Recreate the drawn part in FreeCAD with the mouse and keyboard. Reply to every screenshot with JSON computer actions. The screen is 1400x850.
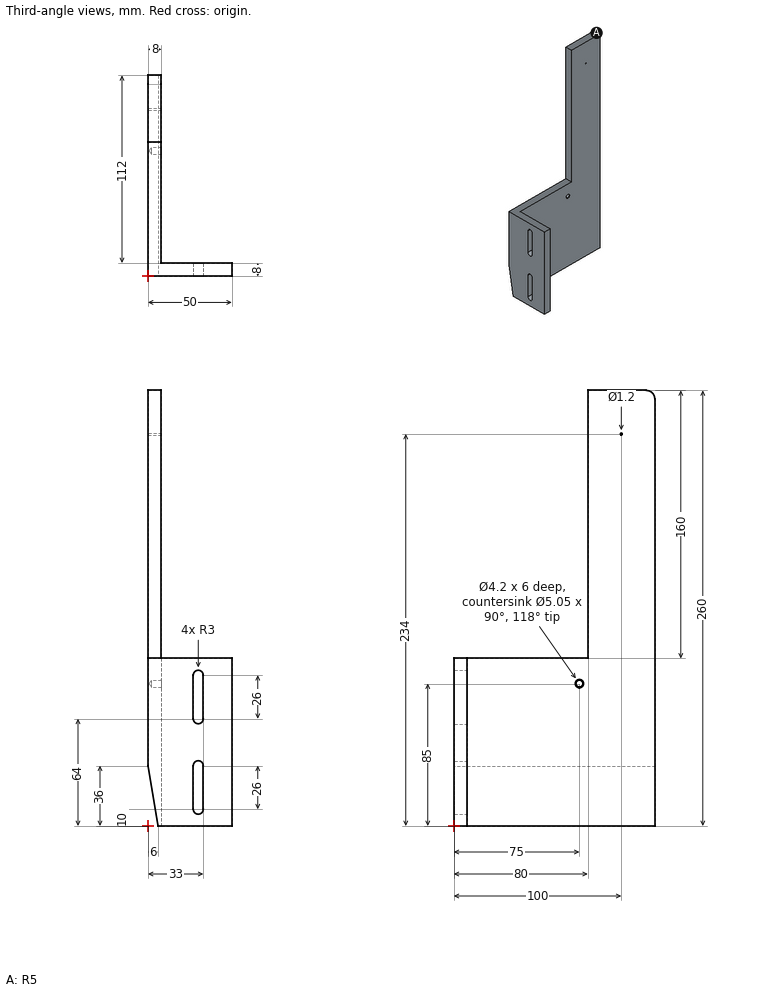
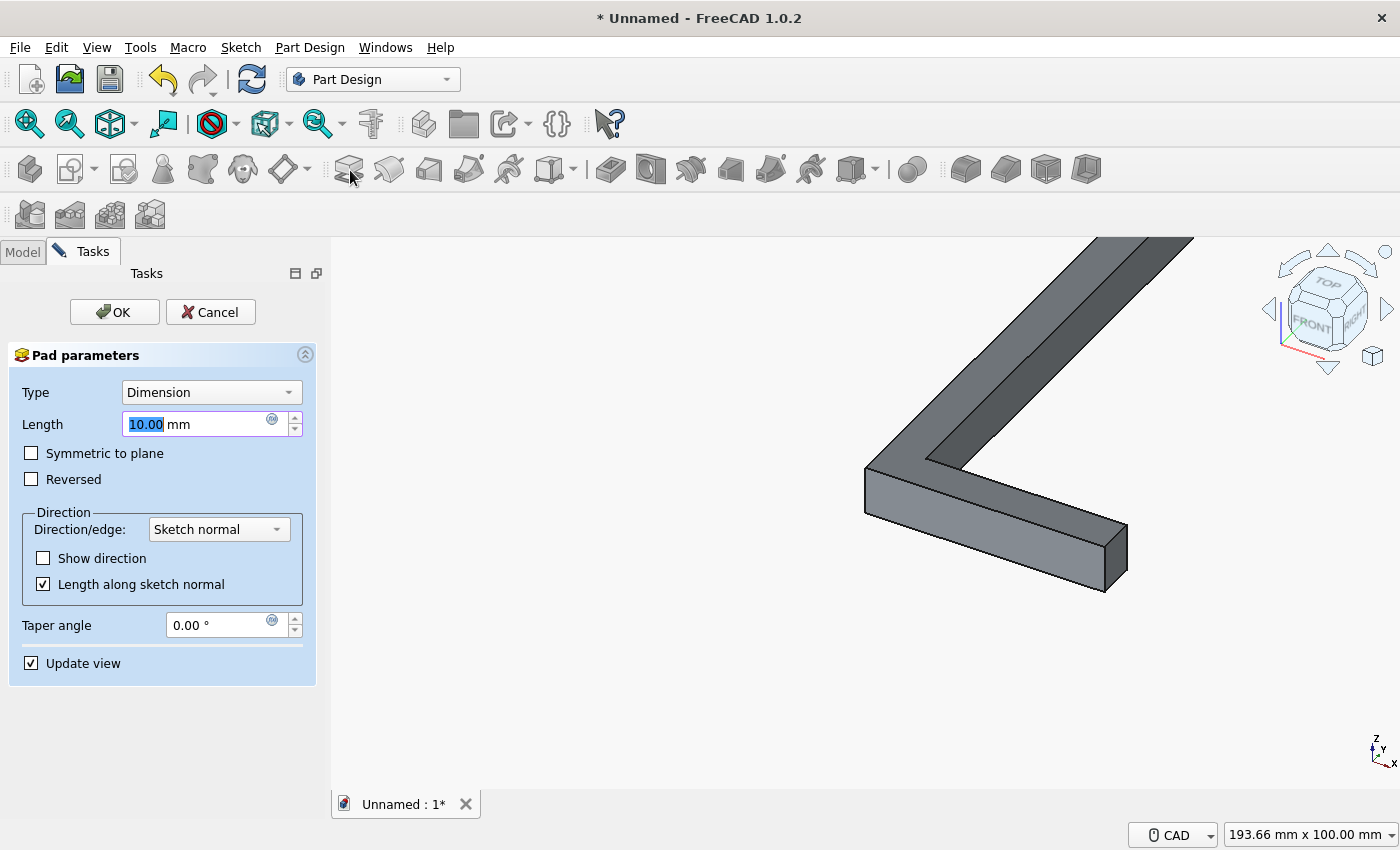
{"action": "type", "text": "260"}
{"action": "key", "text": "Tab"}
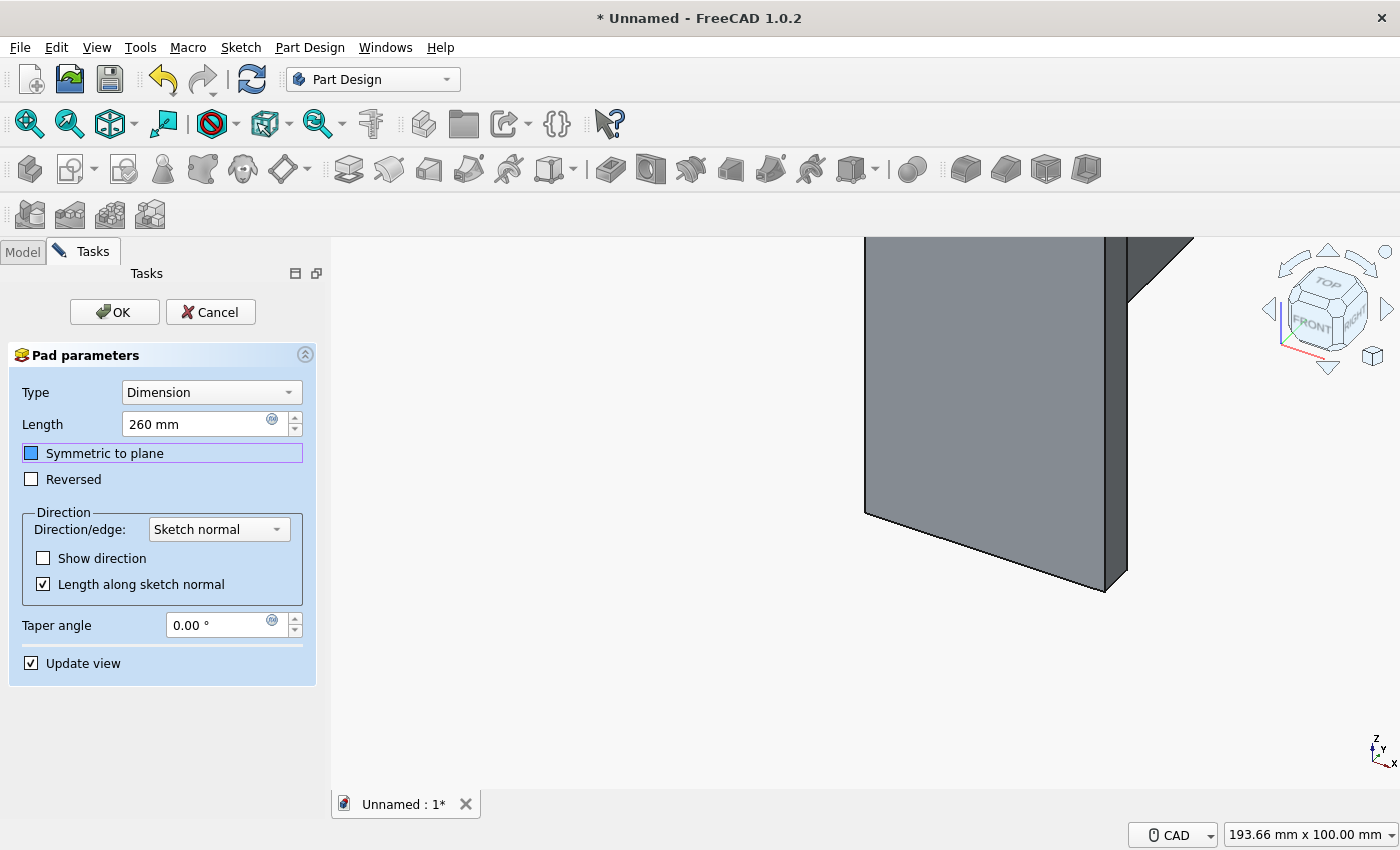
{"action": "left_click", "coordinate": [115, 312]}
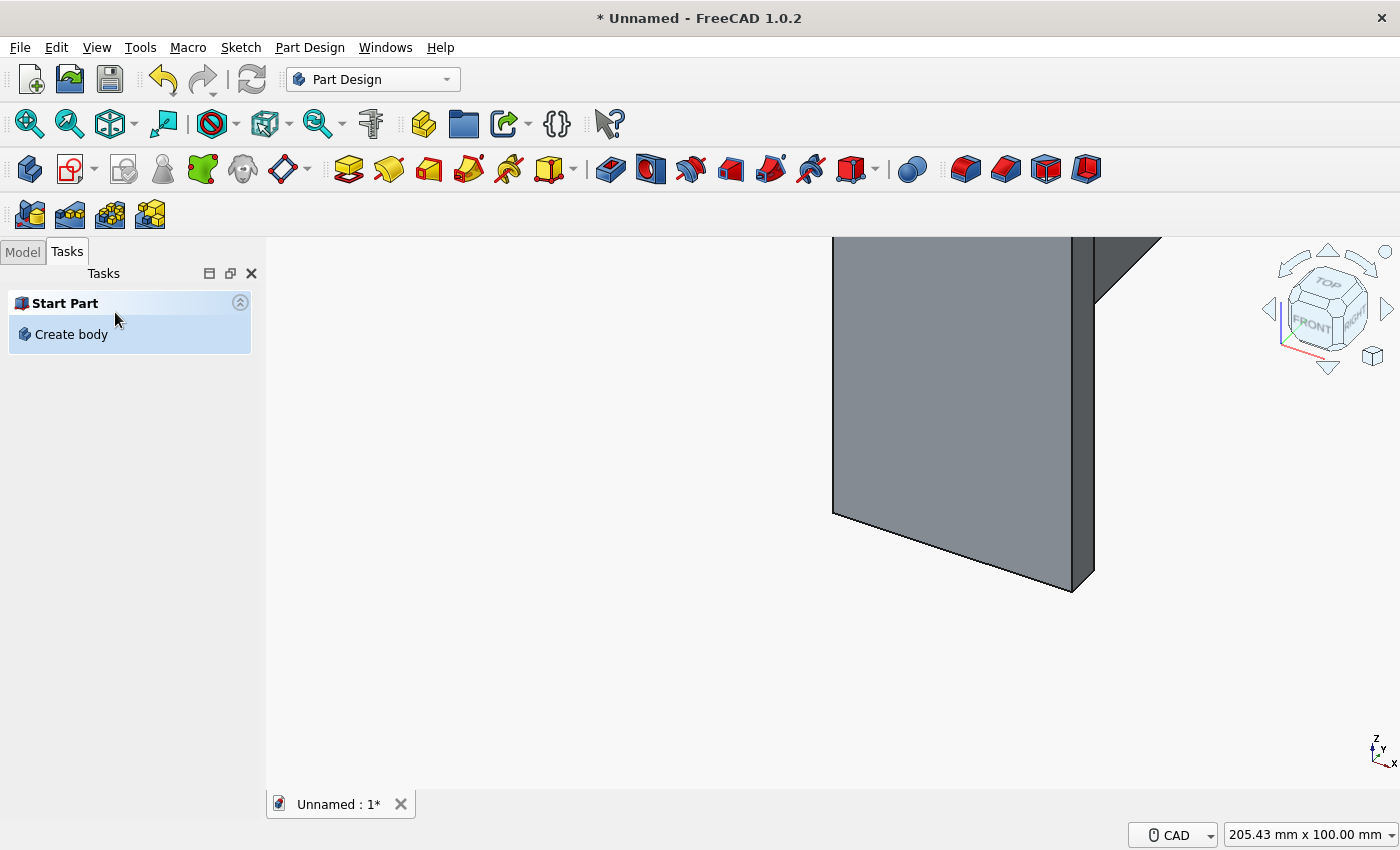
{"action": "left_click", "coordinate": [30, 124]}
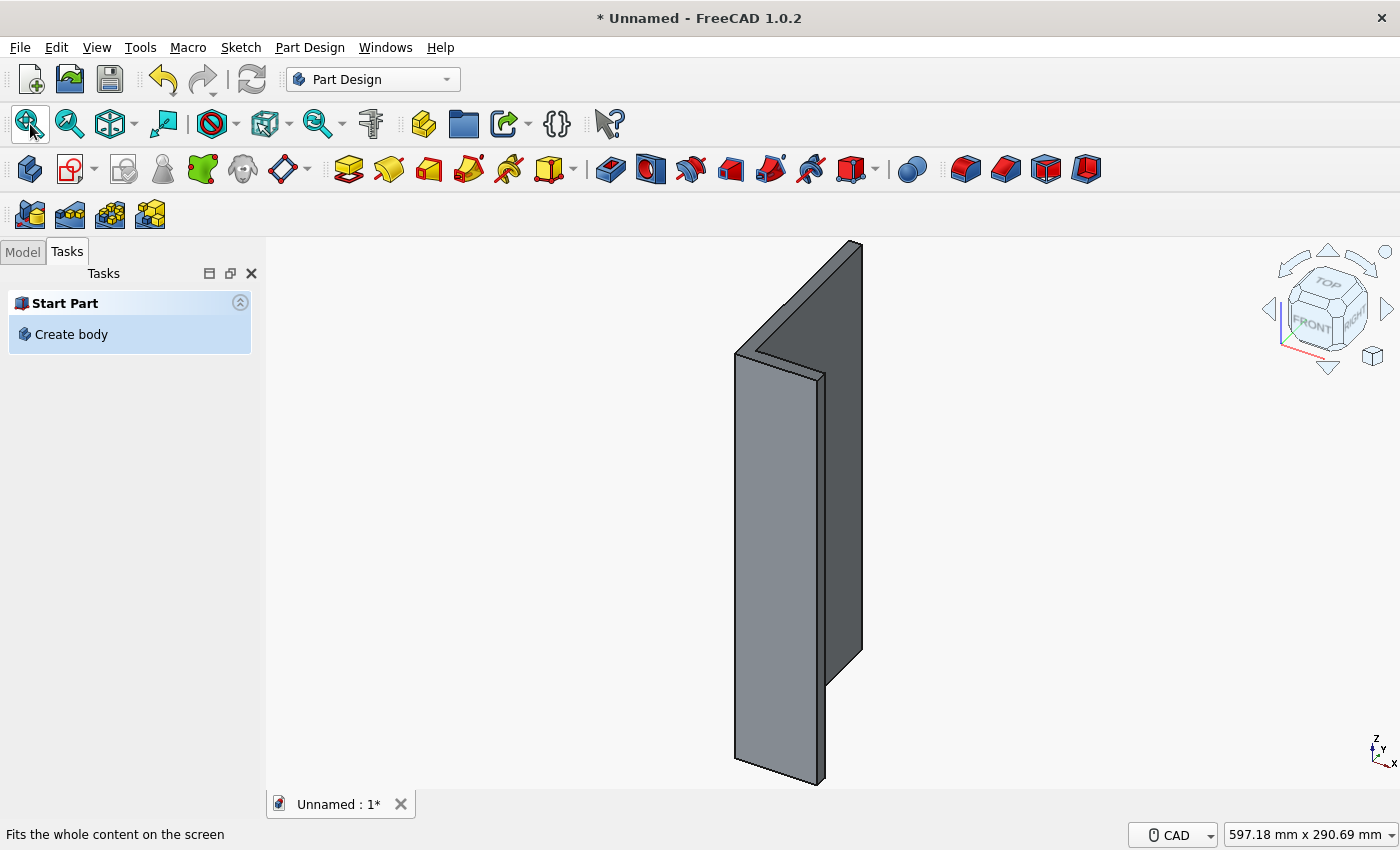
{"action": "key", "text": "0"}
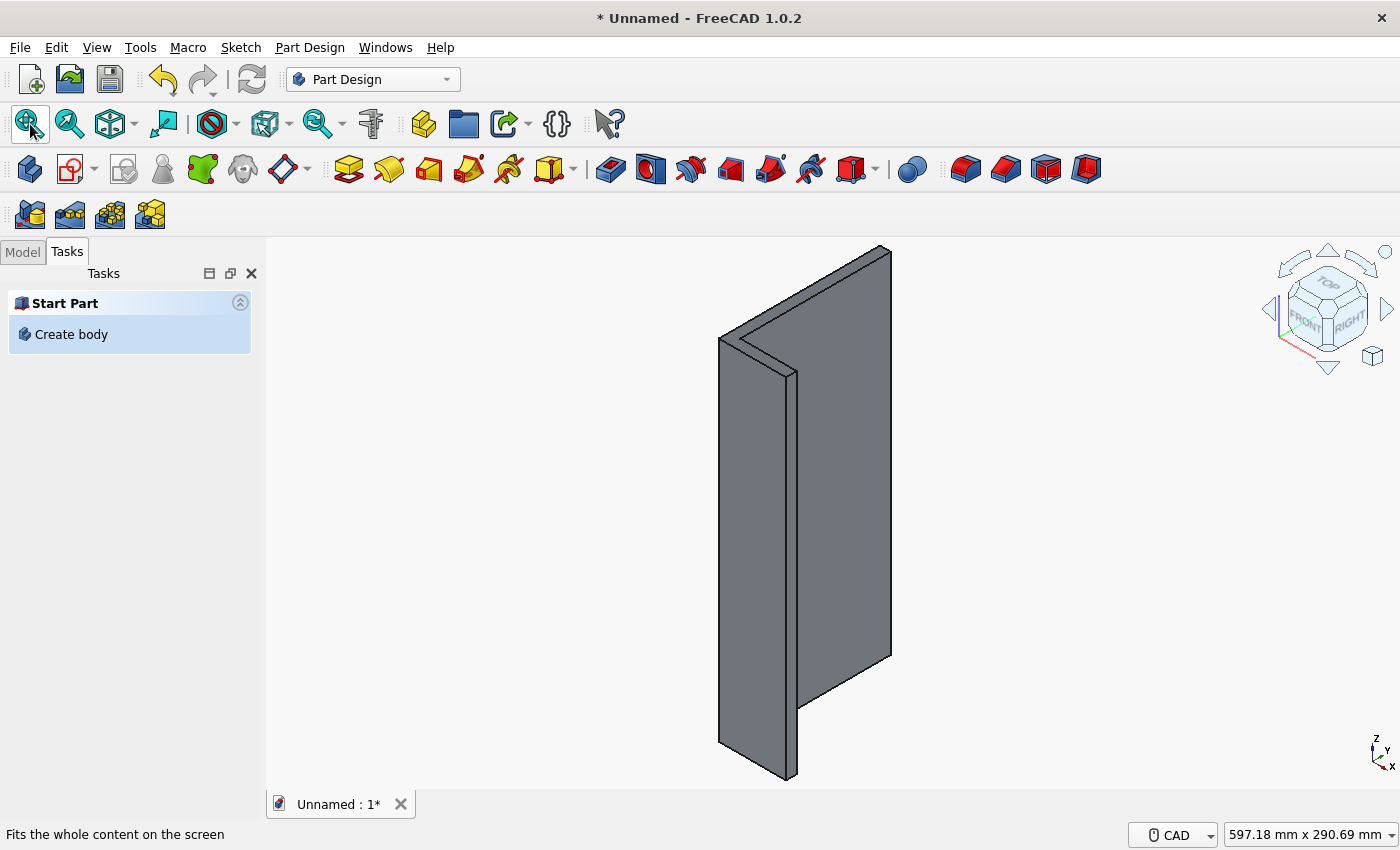
{"action": "key", "text": "3"}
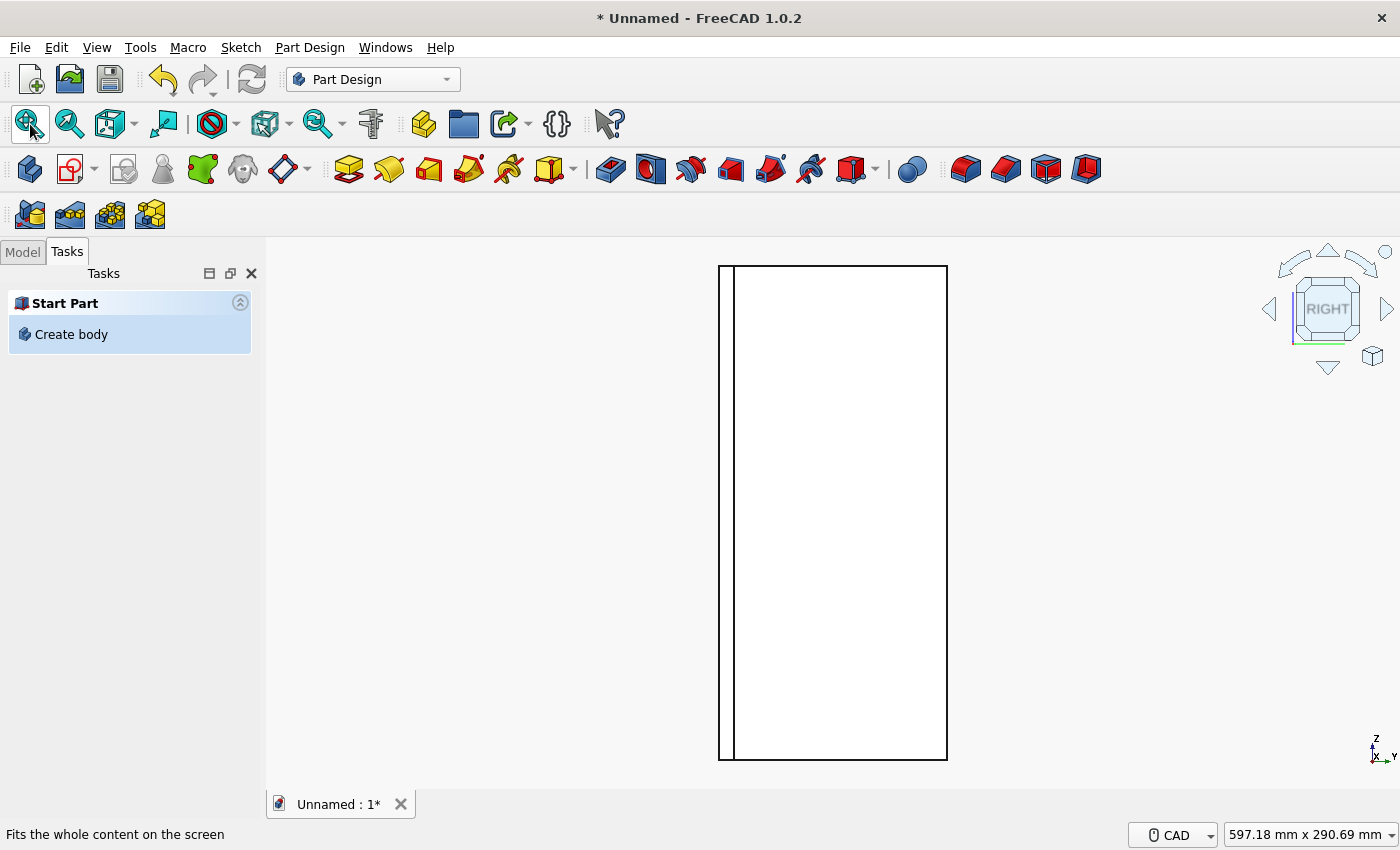
{"action": "key", "text": "2"}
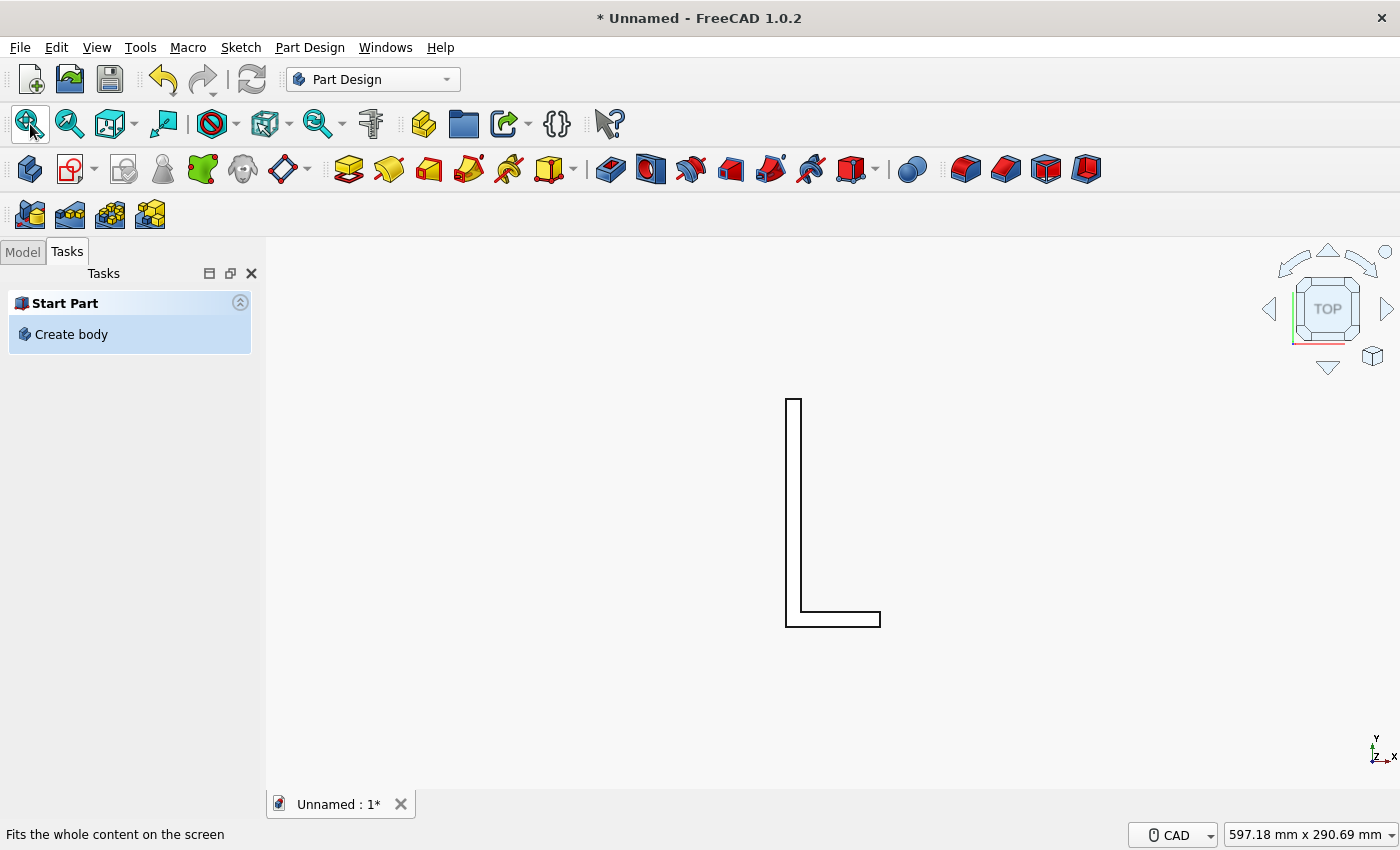
{"action": "left_click", "coordinate": [30, 124]}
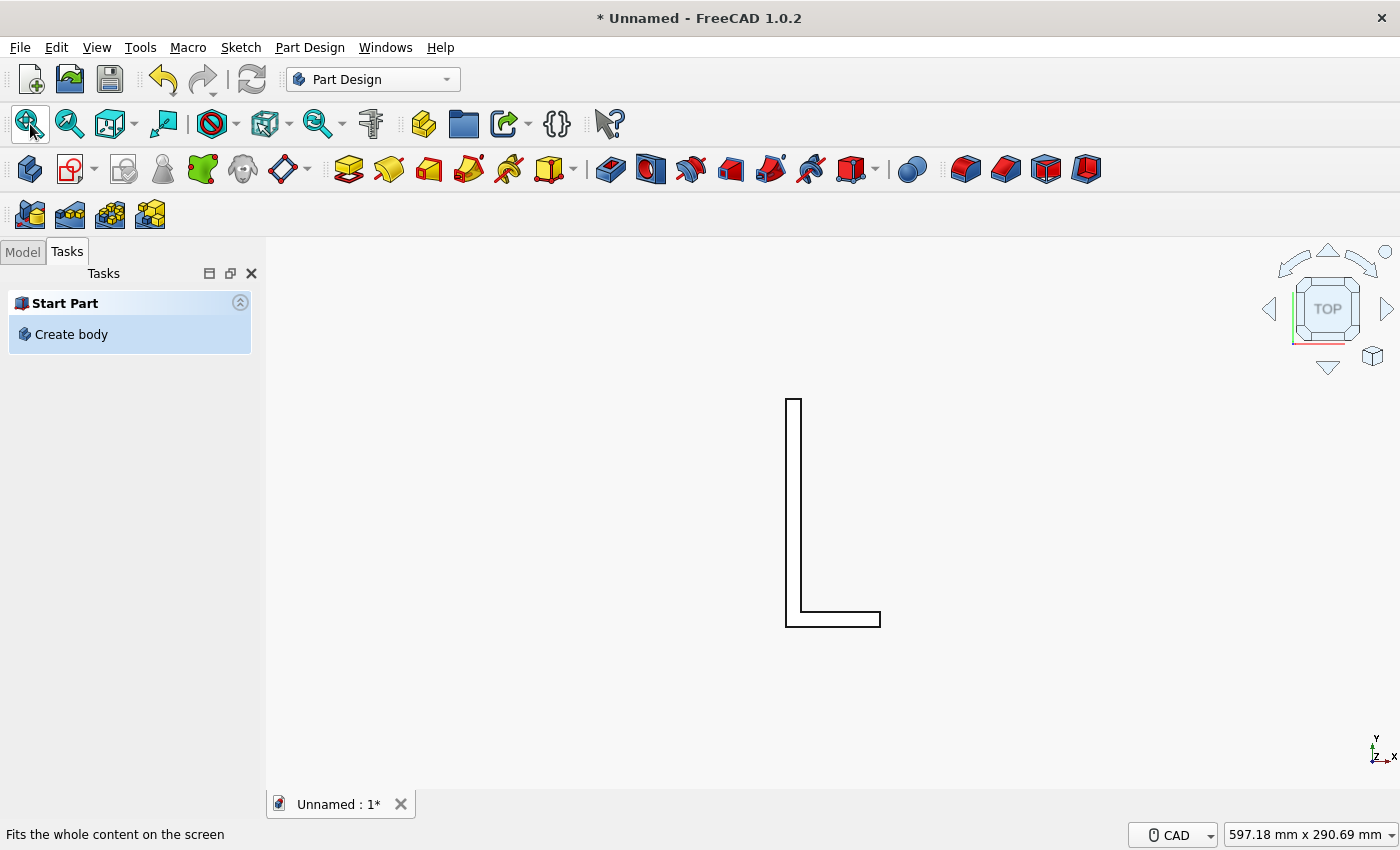
{"action": "left_click", "coordinate": [23, 251]}